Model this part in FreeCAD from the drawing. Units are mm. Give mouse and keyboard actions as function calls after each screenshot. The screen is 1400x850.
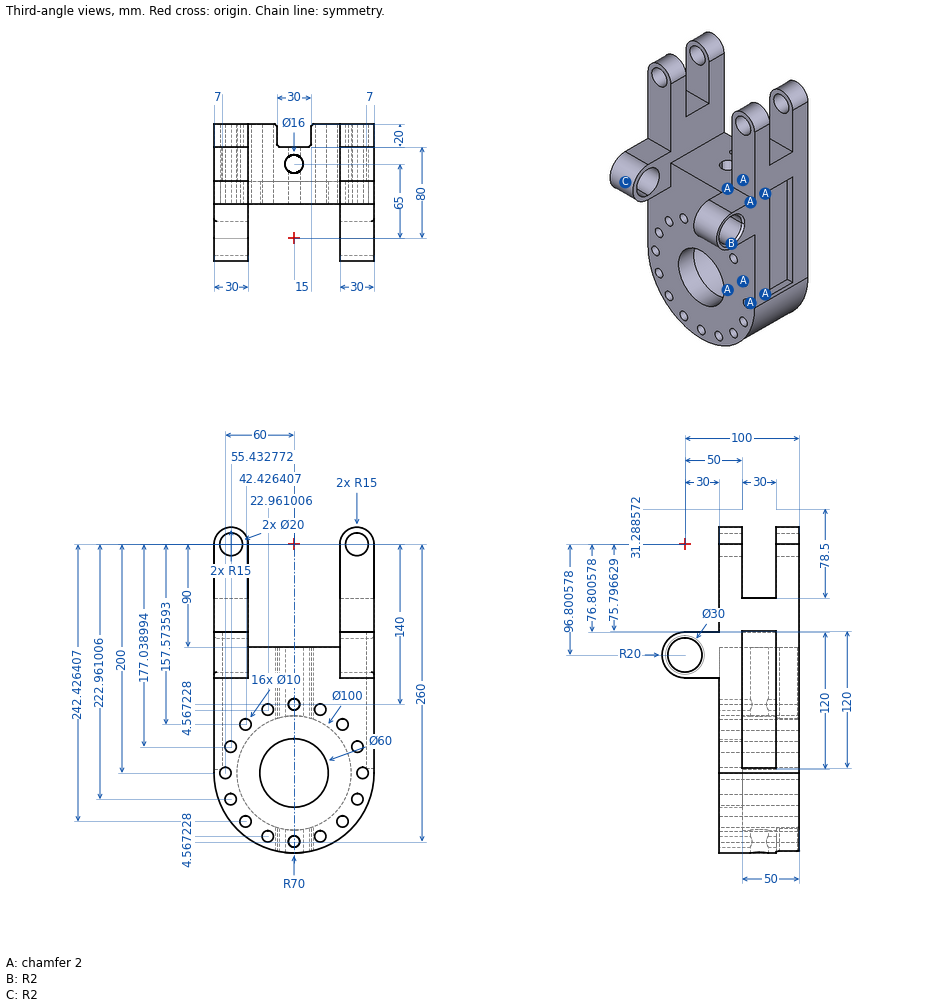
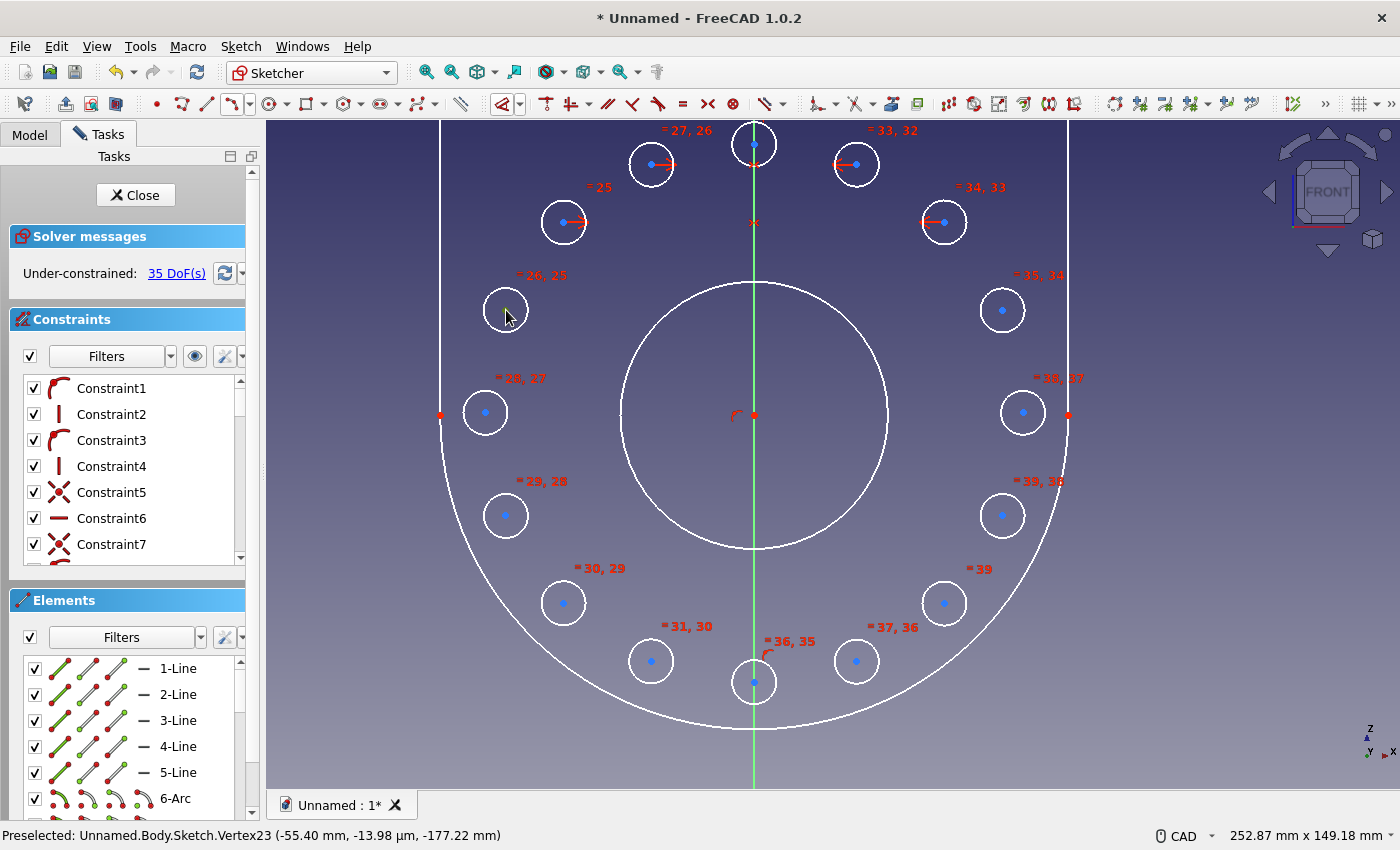
click(1003, 310)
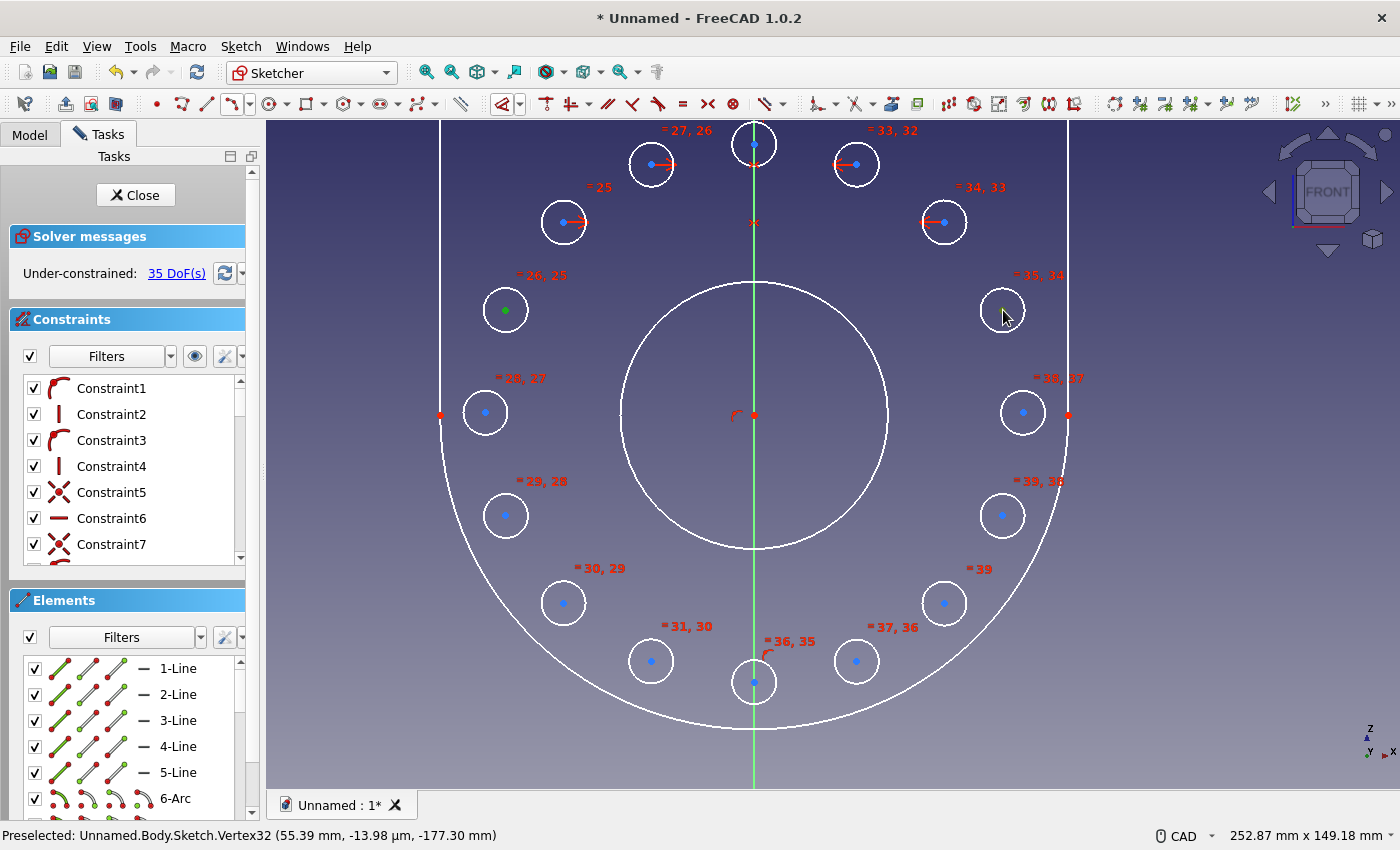
click(754, 630)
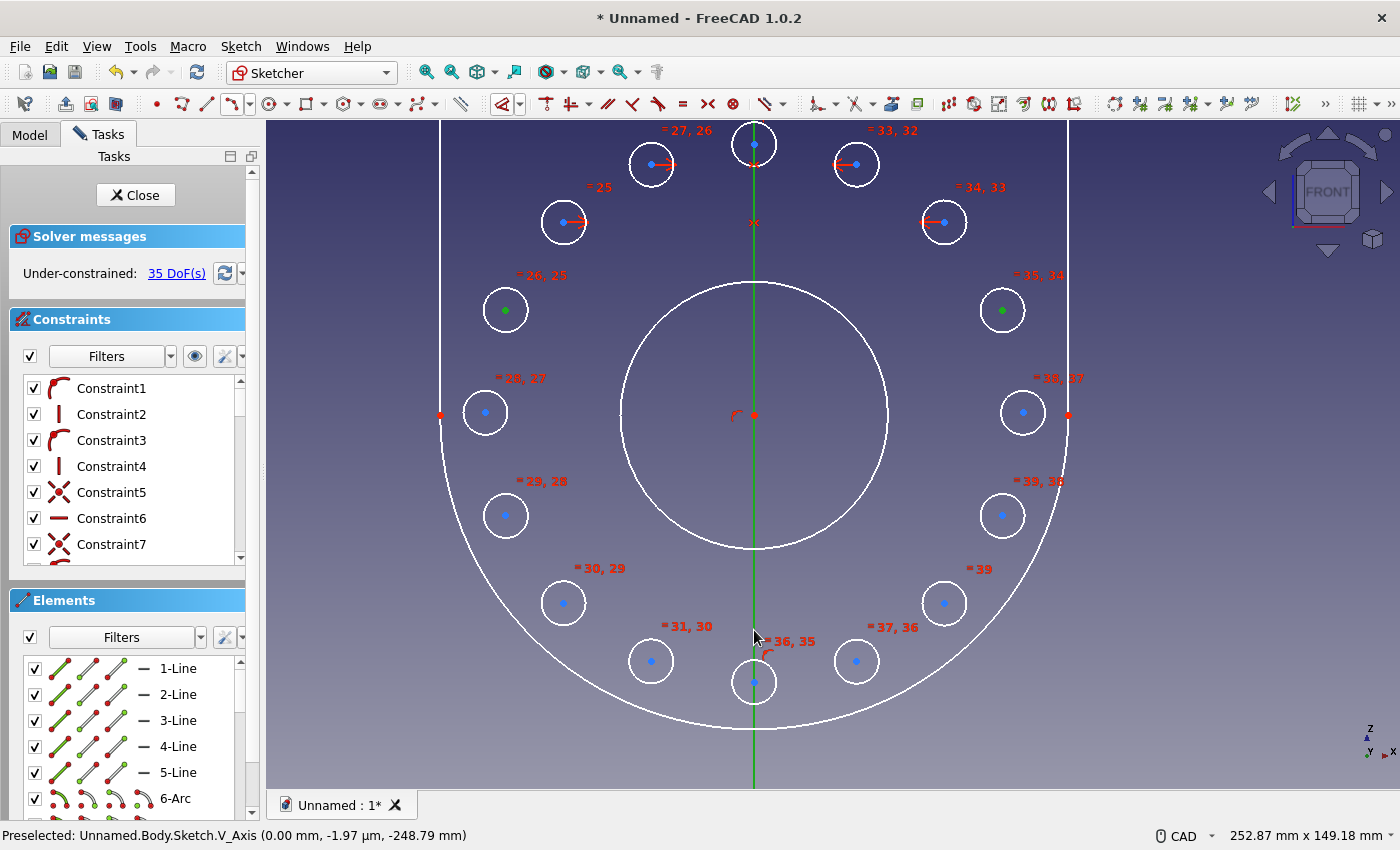
key(s)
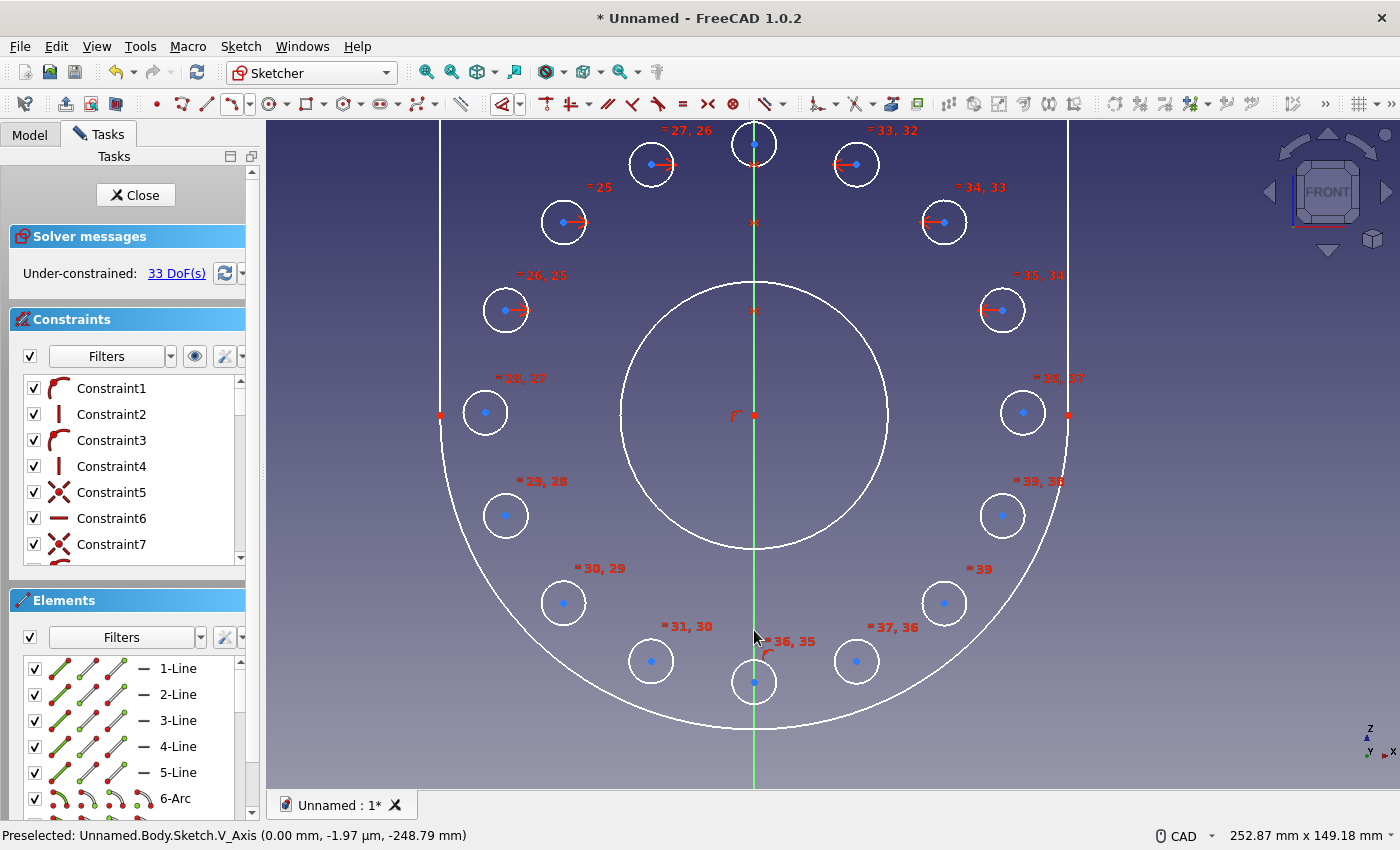
click(651, 661)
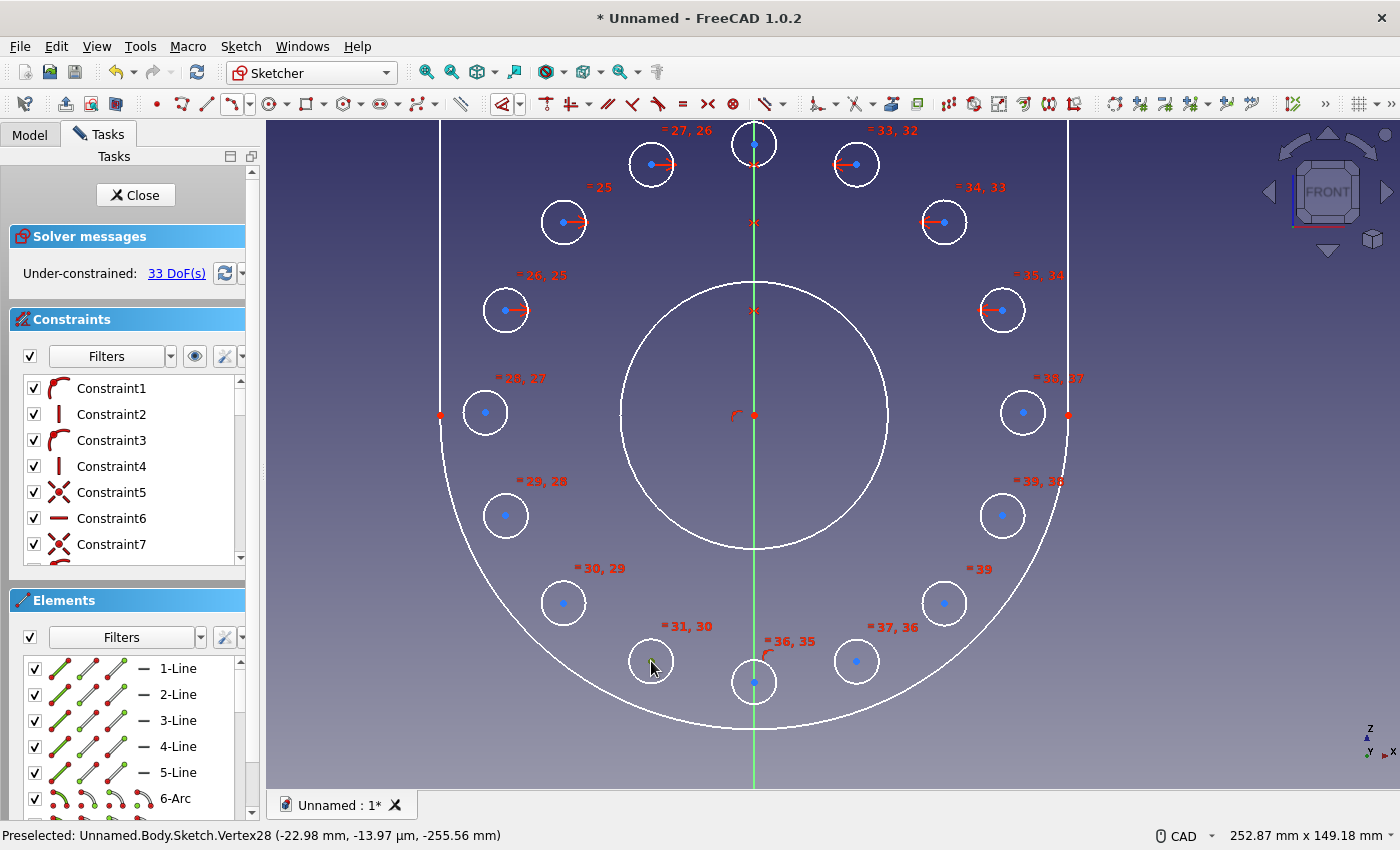
click(857, 662)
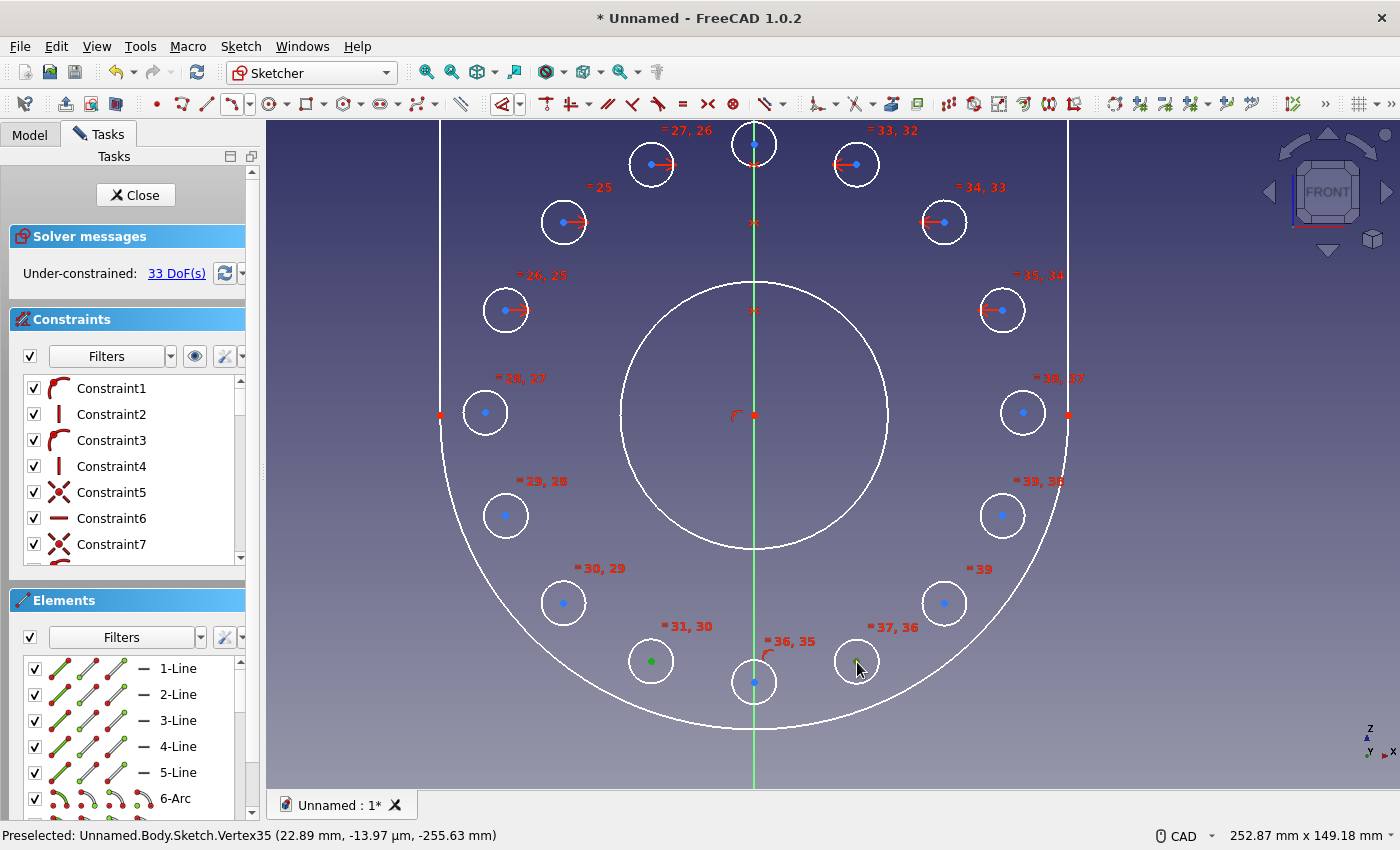
click(754, 630)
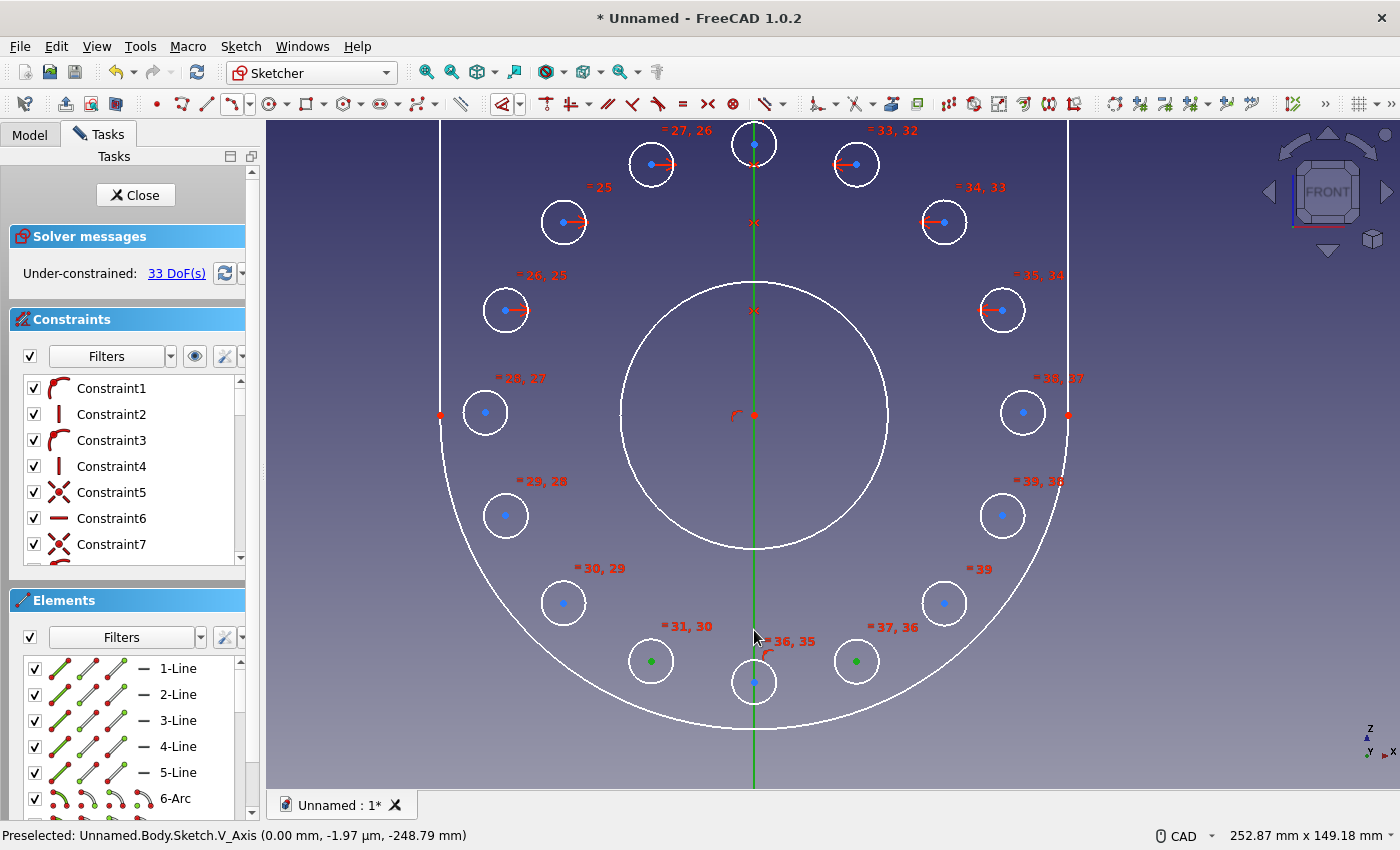
key(s)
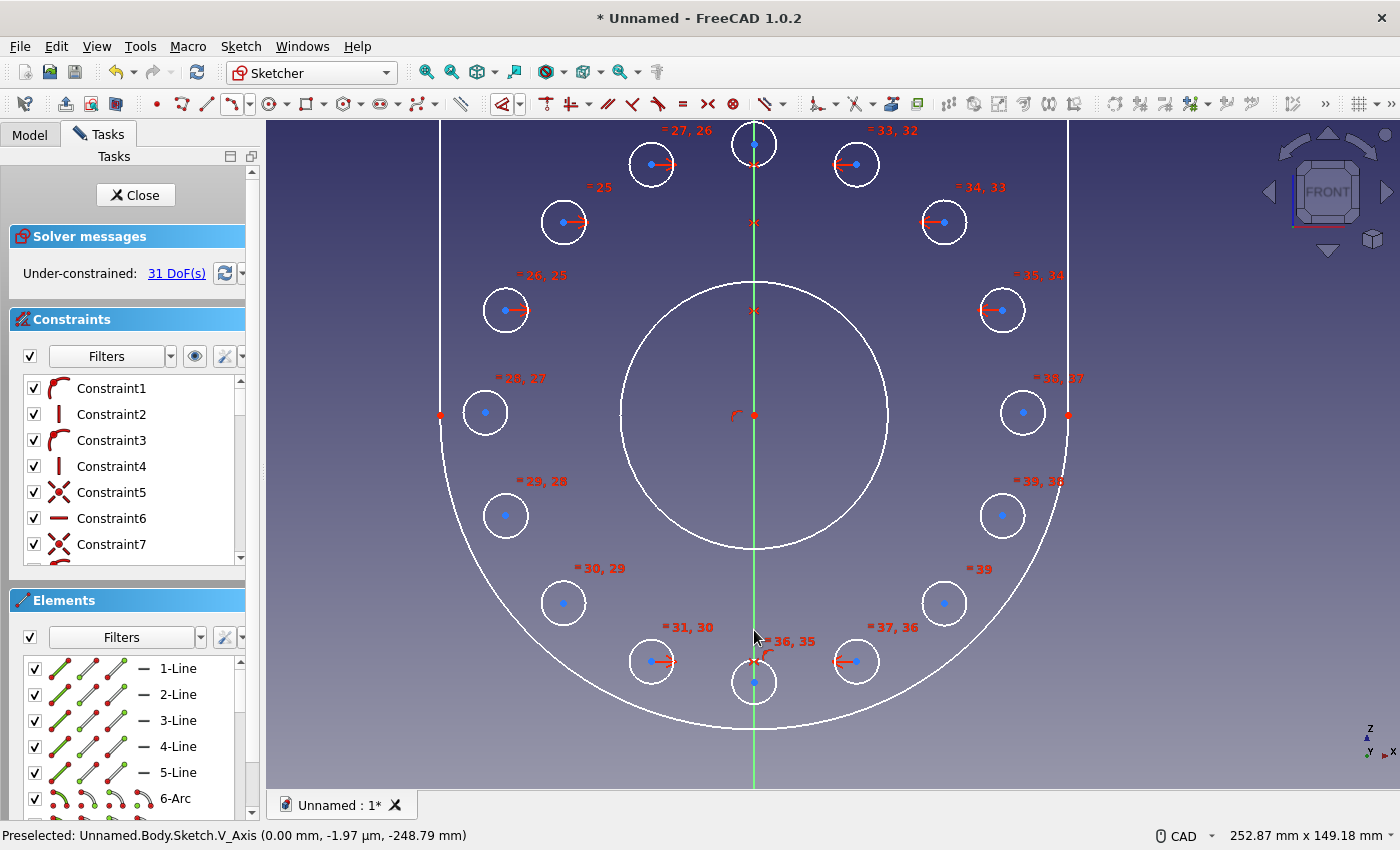
click(486, 413)